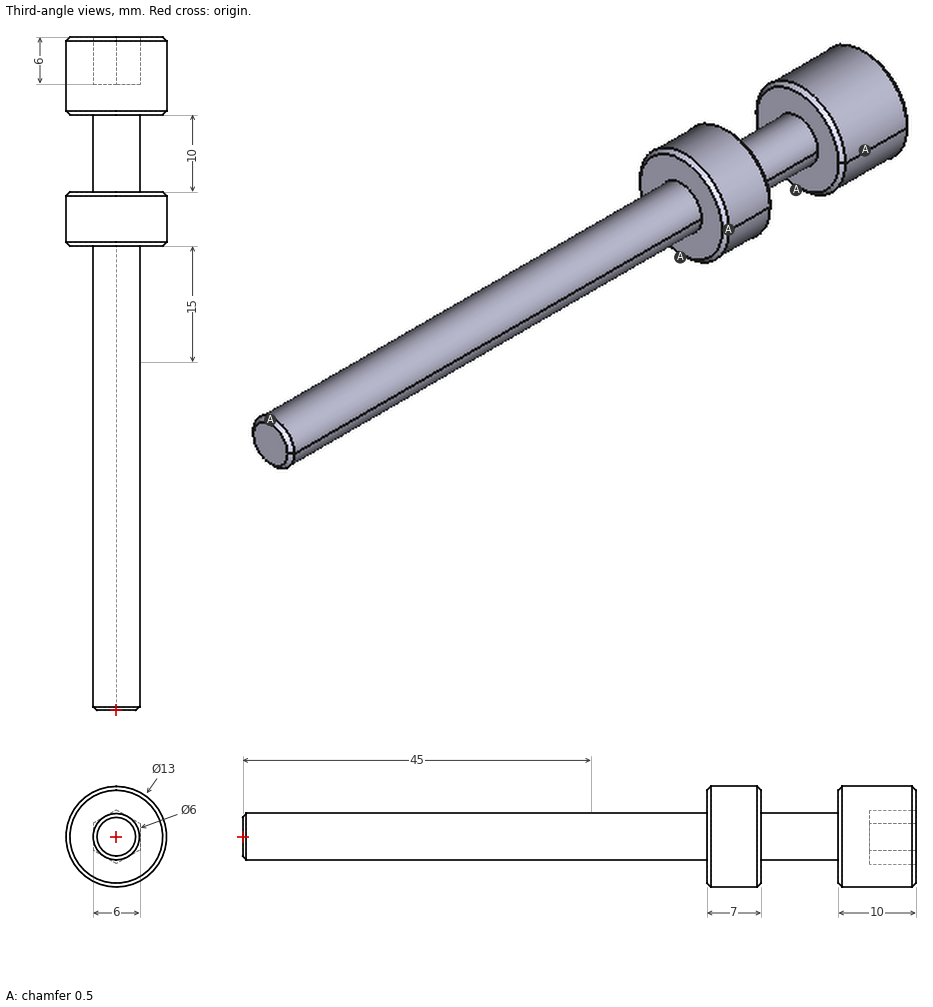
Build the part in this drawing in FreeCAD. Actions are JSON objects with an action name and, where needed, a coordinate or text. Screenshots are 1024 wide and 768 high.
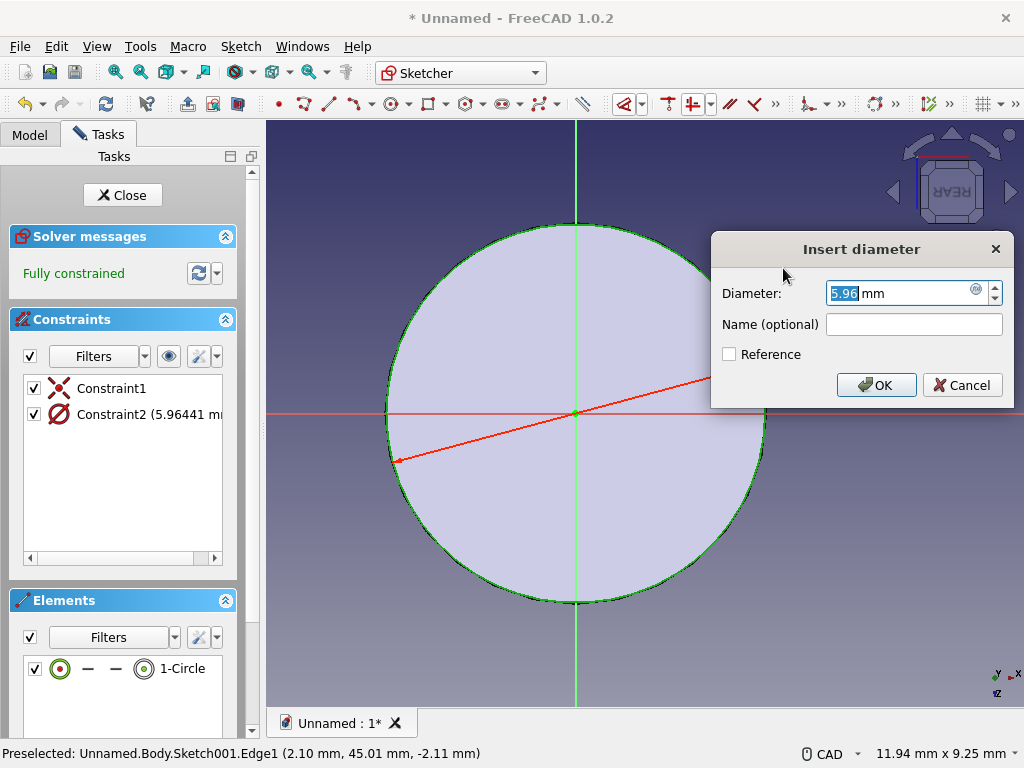
{"action": "type", "text": "6"}
{"action": "key", "text": "Return"}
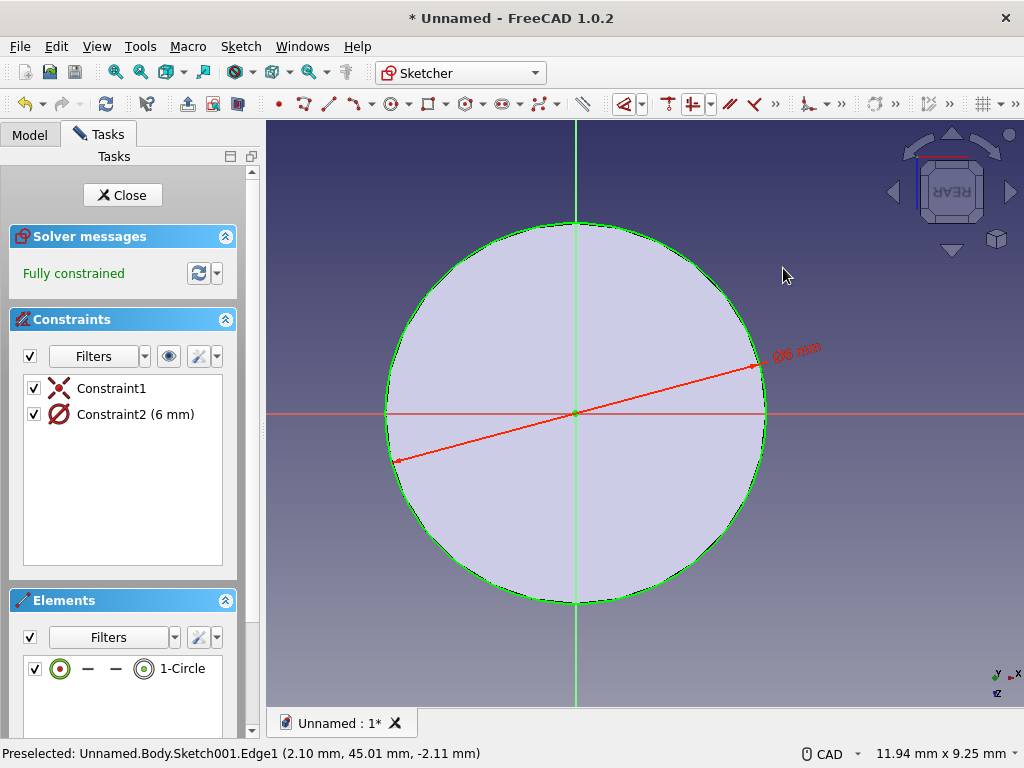
{"action": "left_click", "coordinate": [123, 195]}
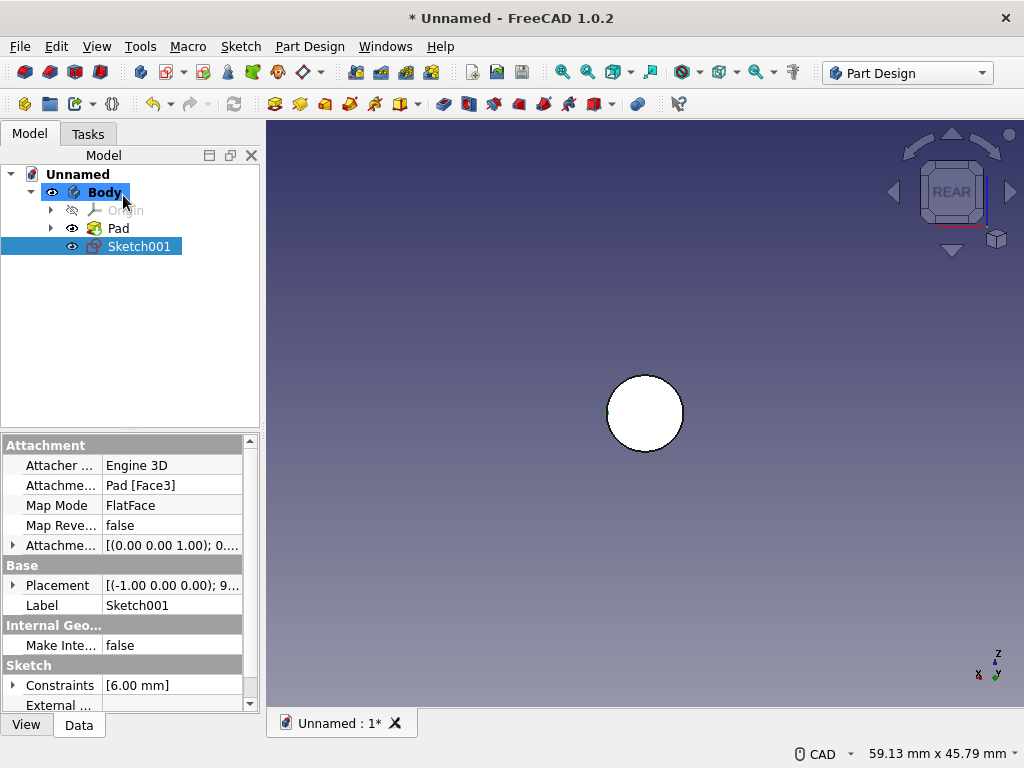
{"action": "left_click", "coordinate": [275, 104]}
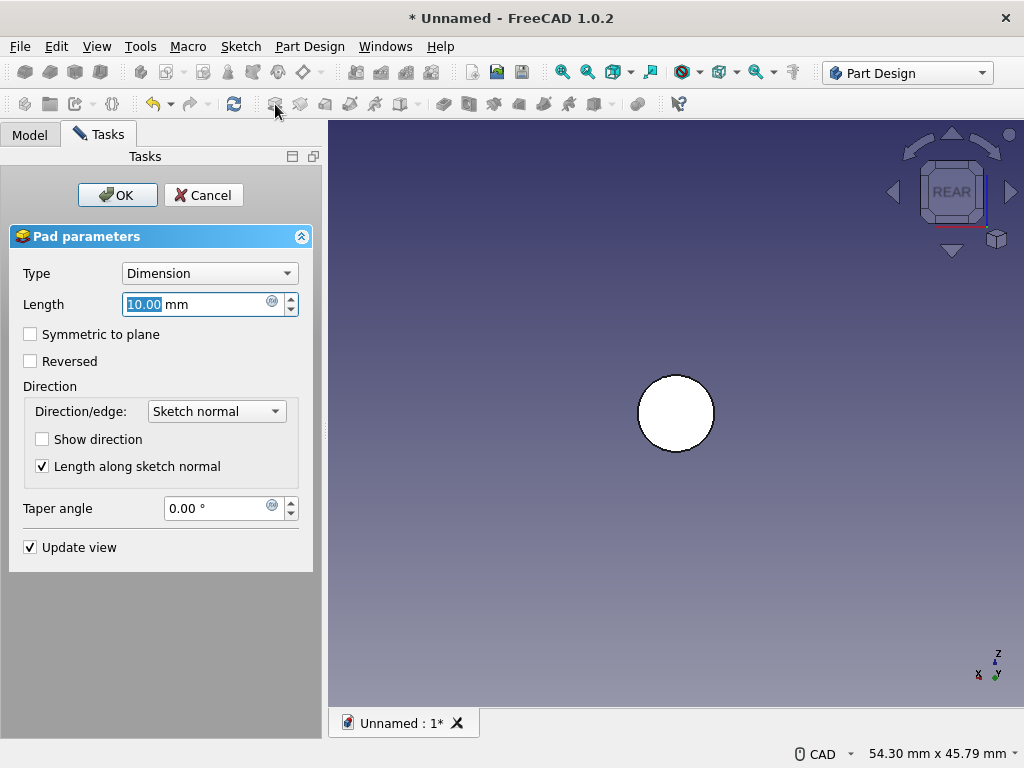
{"action": "type", "text": "15"}
{"action": "key", "text": "Tab"}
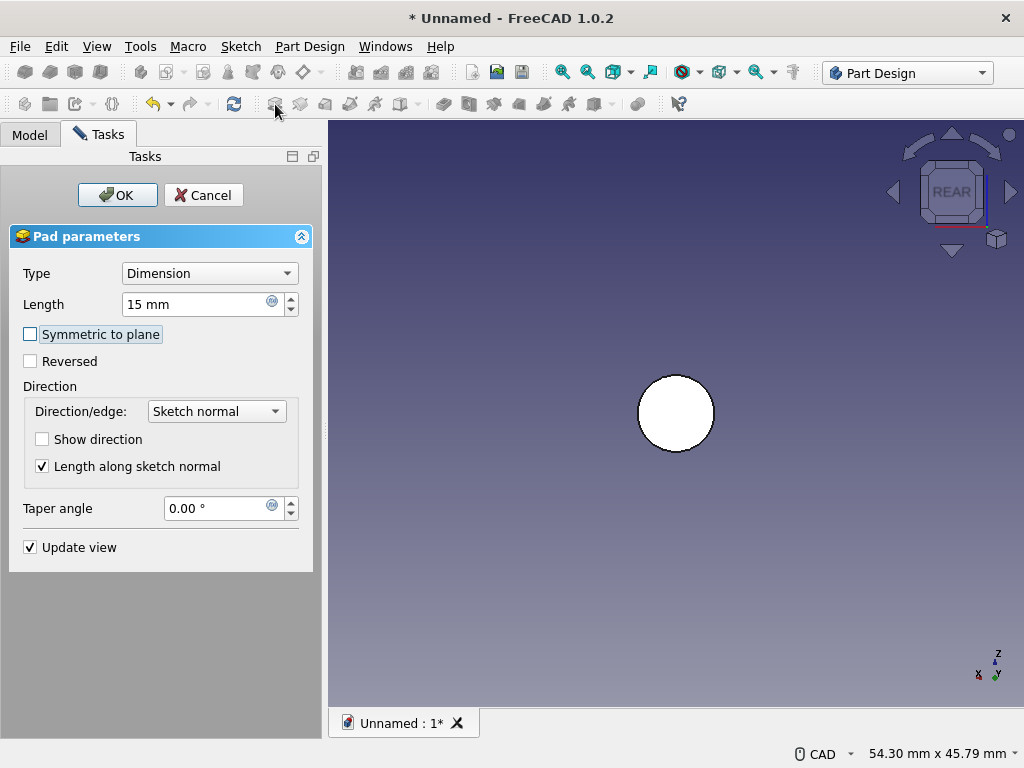
{"action": "left_click", "coordinate": [118, 195]}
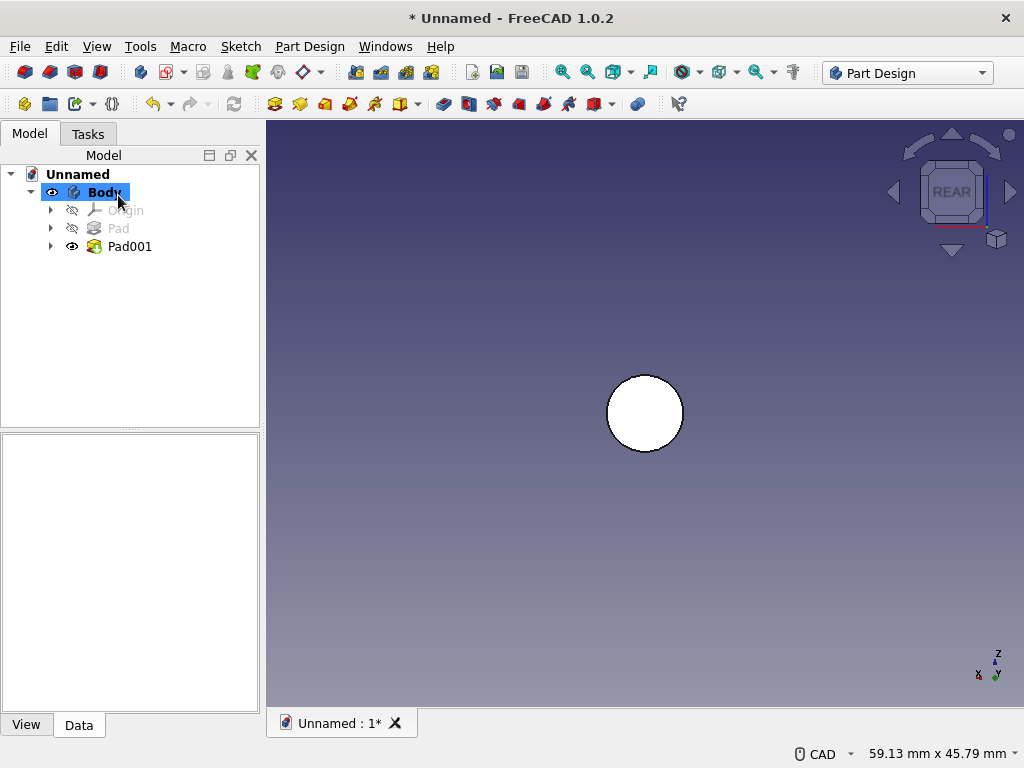
{"action": "left_click", "coordinate": [563, 72]}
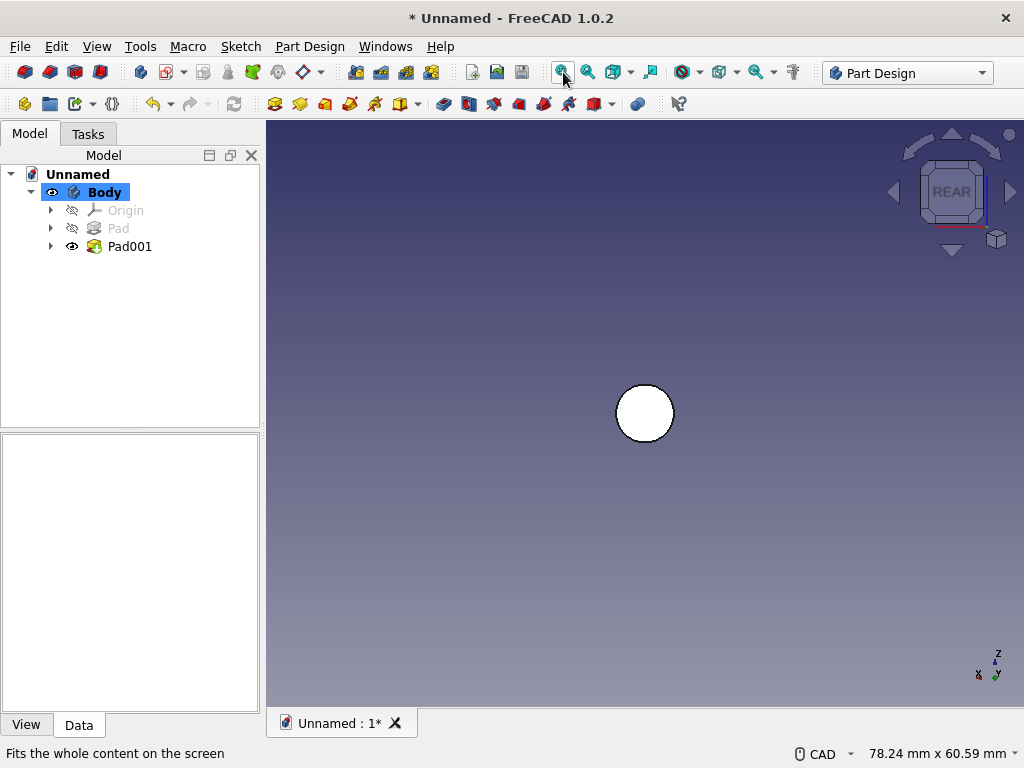
{"action": "left_click", "coordinate": [645, 412]}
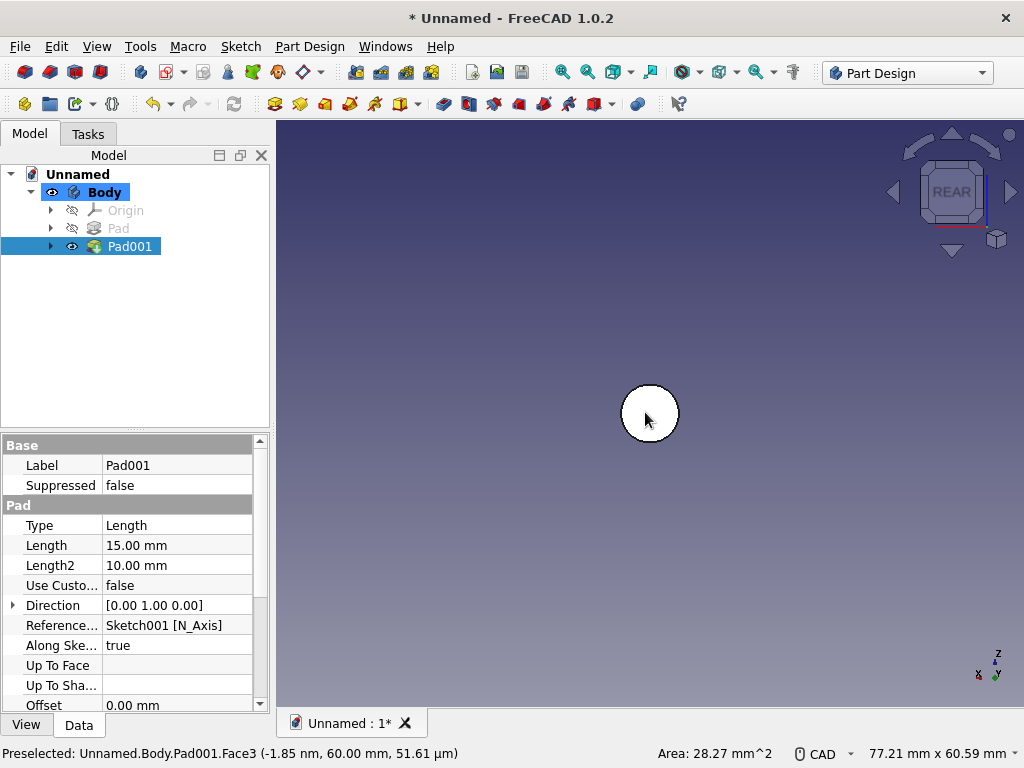
{"action": "left_click", "coordinate": [166, 72]}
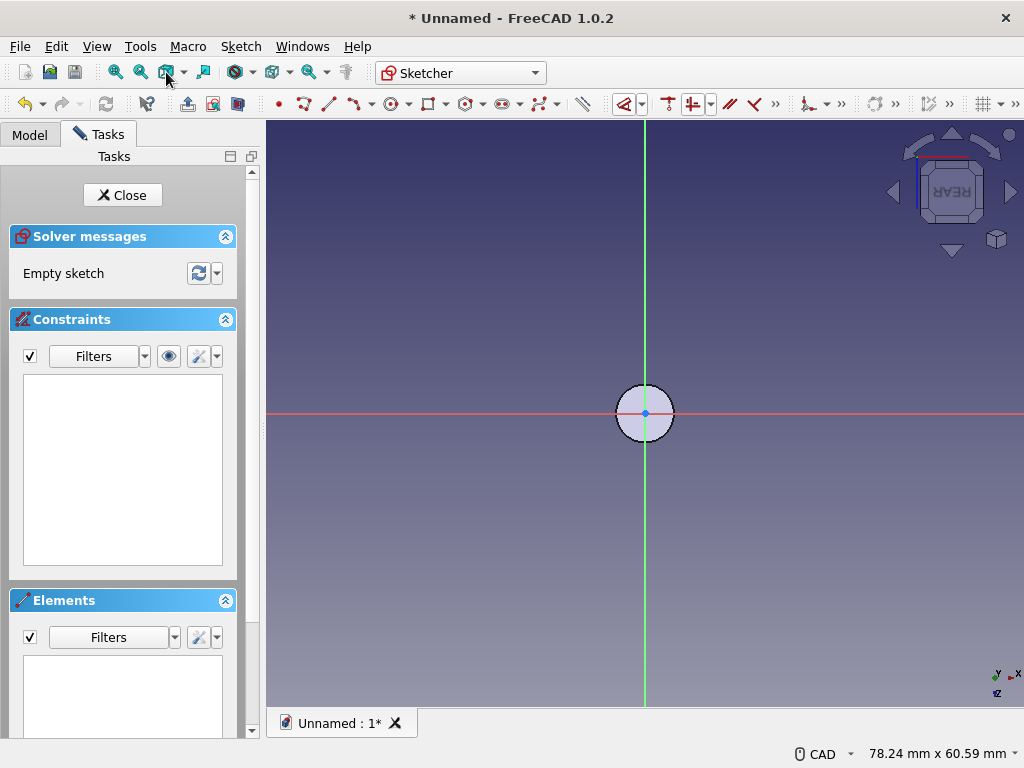
{"action": "scroll", "coordinate": [685, 413], "scroll_direction": "up", "scroll_amount": 5}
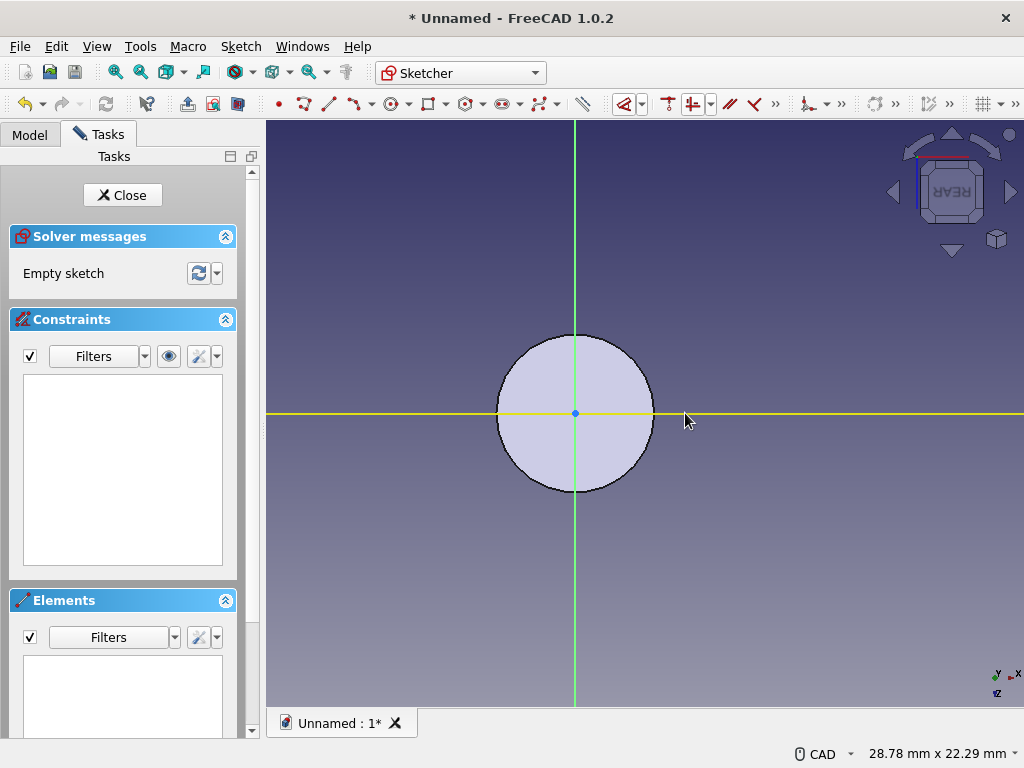
{"action": "key", "text": "g c"}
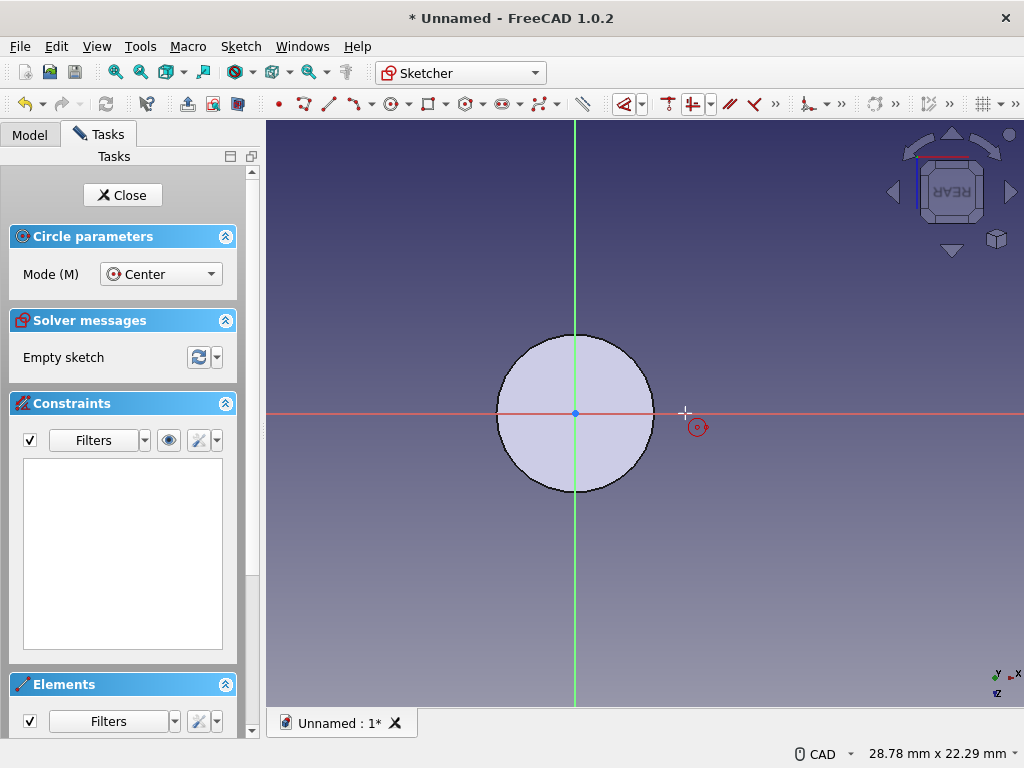
{"action": "left_click", "coordinate": [575, 413]}
{"action": "left_click", "coordinate": [696, 292]}
{"action": "key", "text": "Escape"}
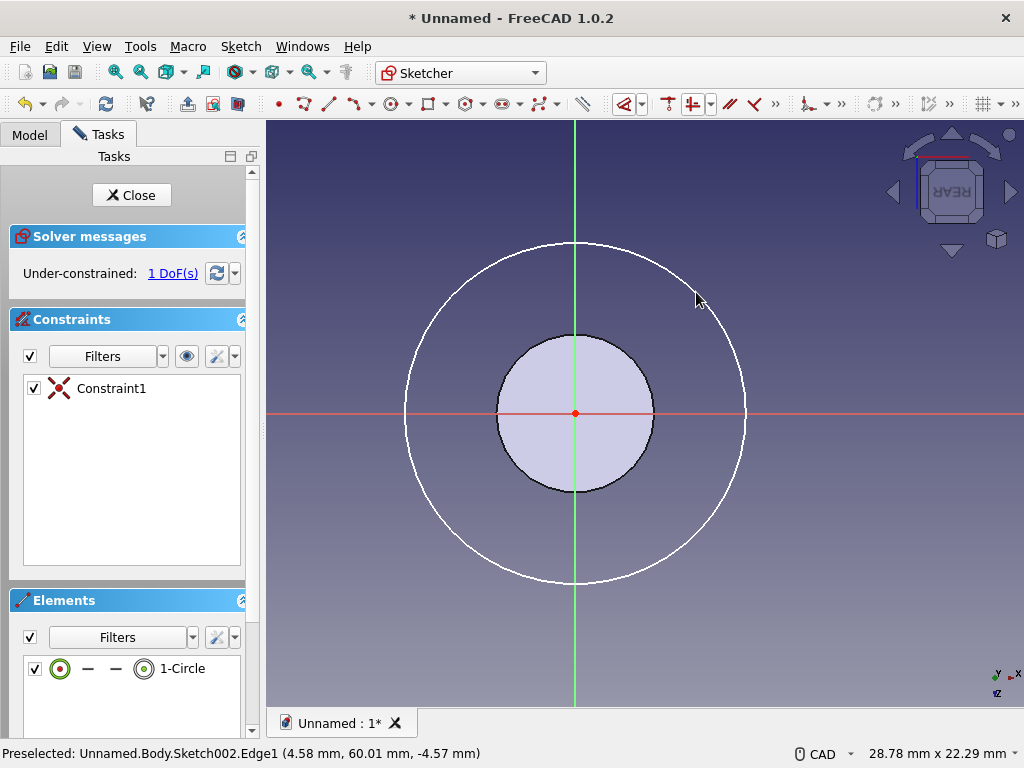
{"action": "left_click", "coordinate": [696, 293]}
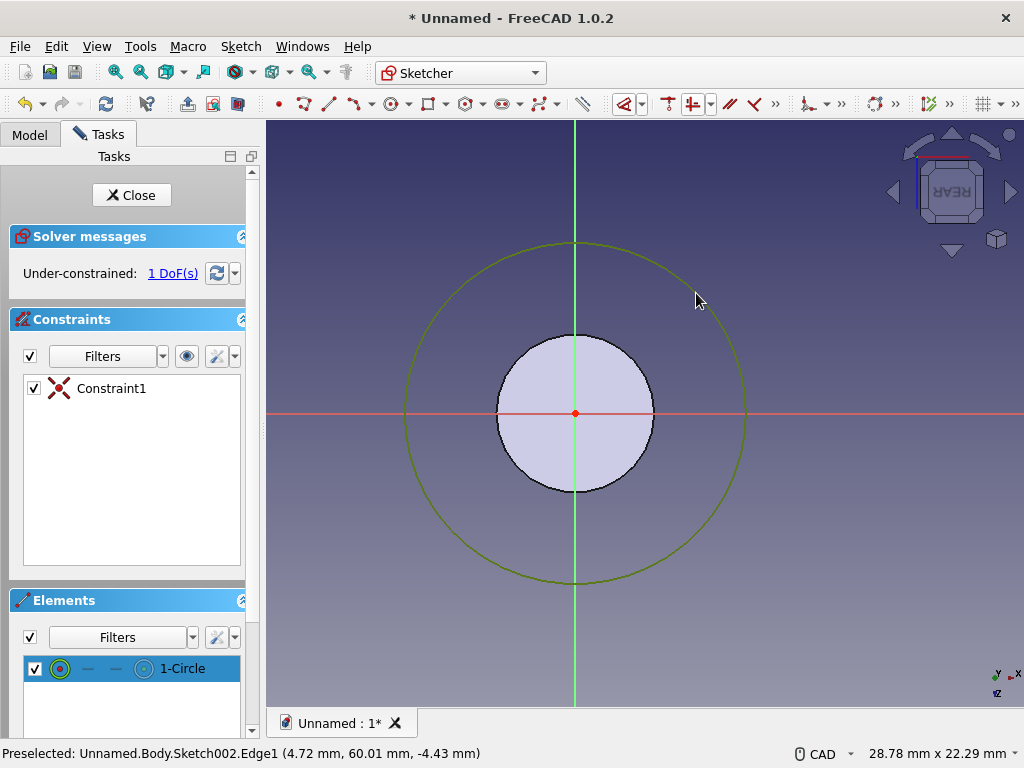
{"action": "key", "text": "k o"}